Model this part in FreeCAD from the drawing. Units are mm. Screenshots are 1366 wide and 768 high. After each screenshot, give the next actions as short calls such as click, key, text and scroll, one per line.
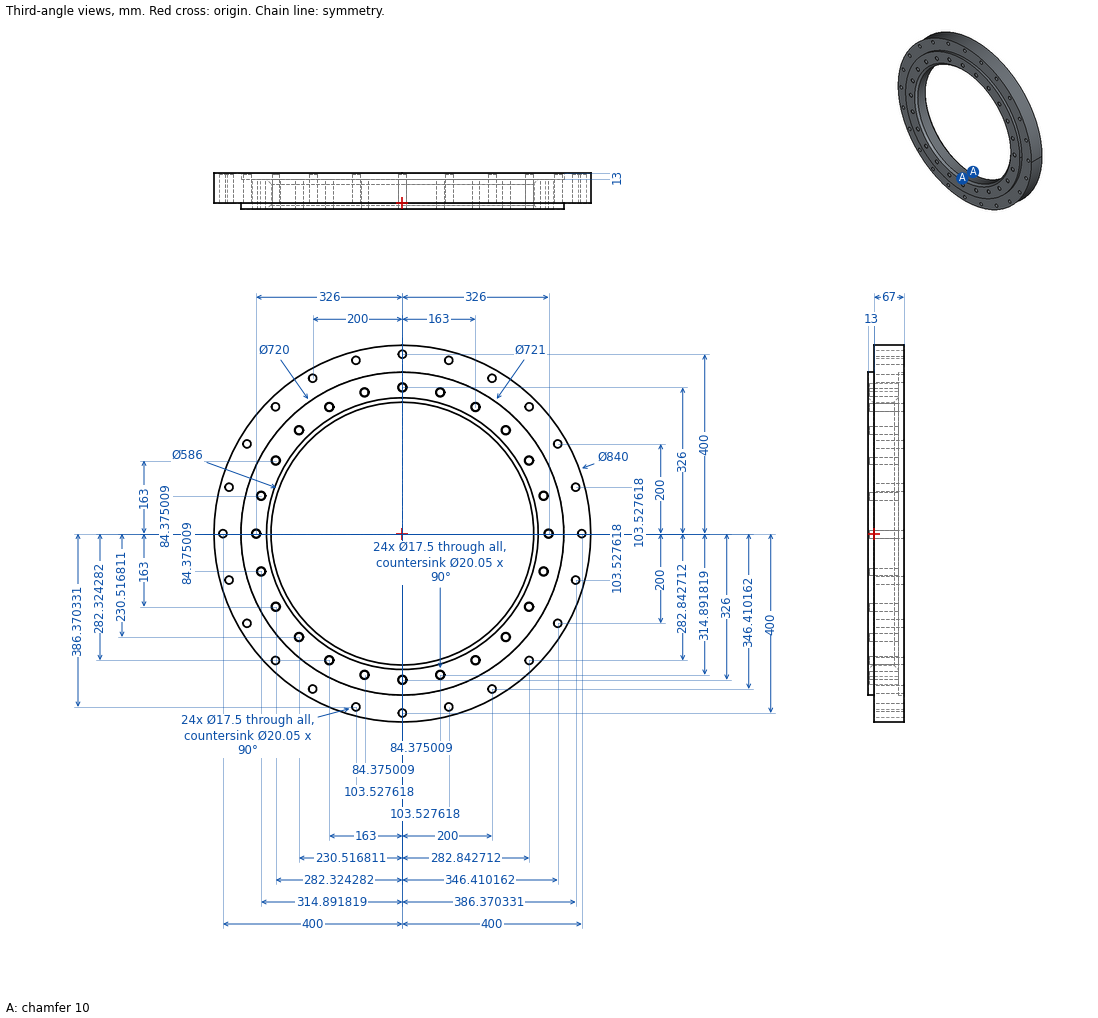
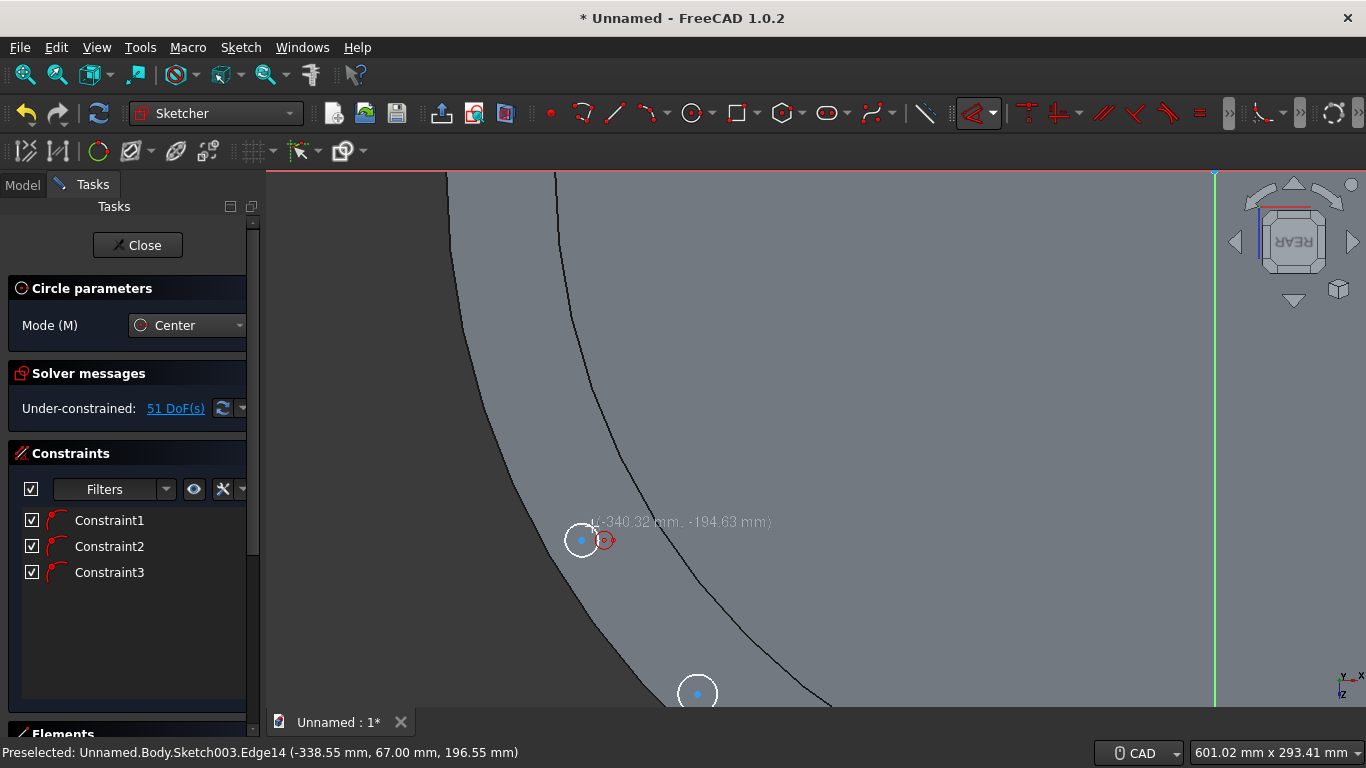
scroll(508, 360, up, 2)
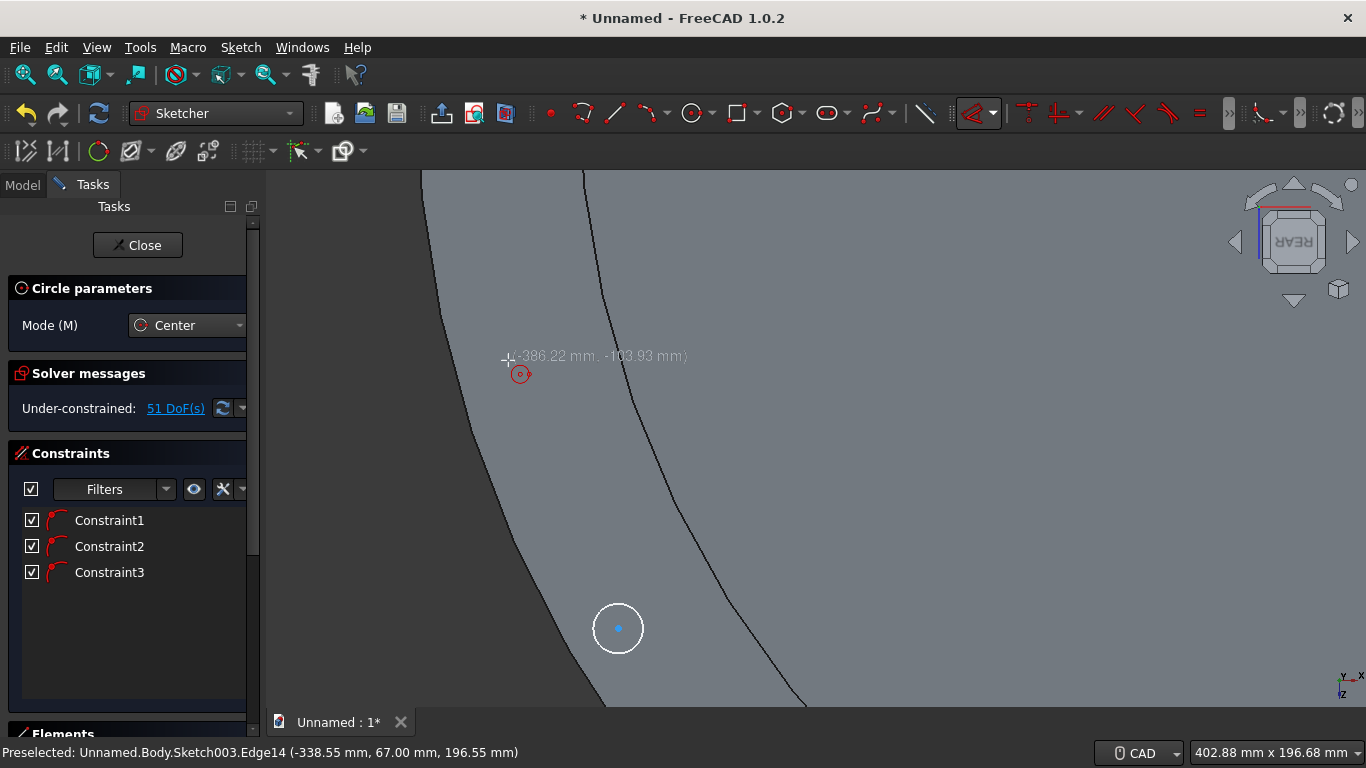
scroll(586, 510, down, 9)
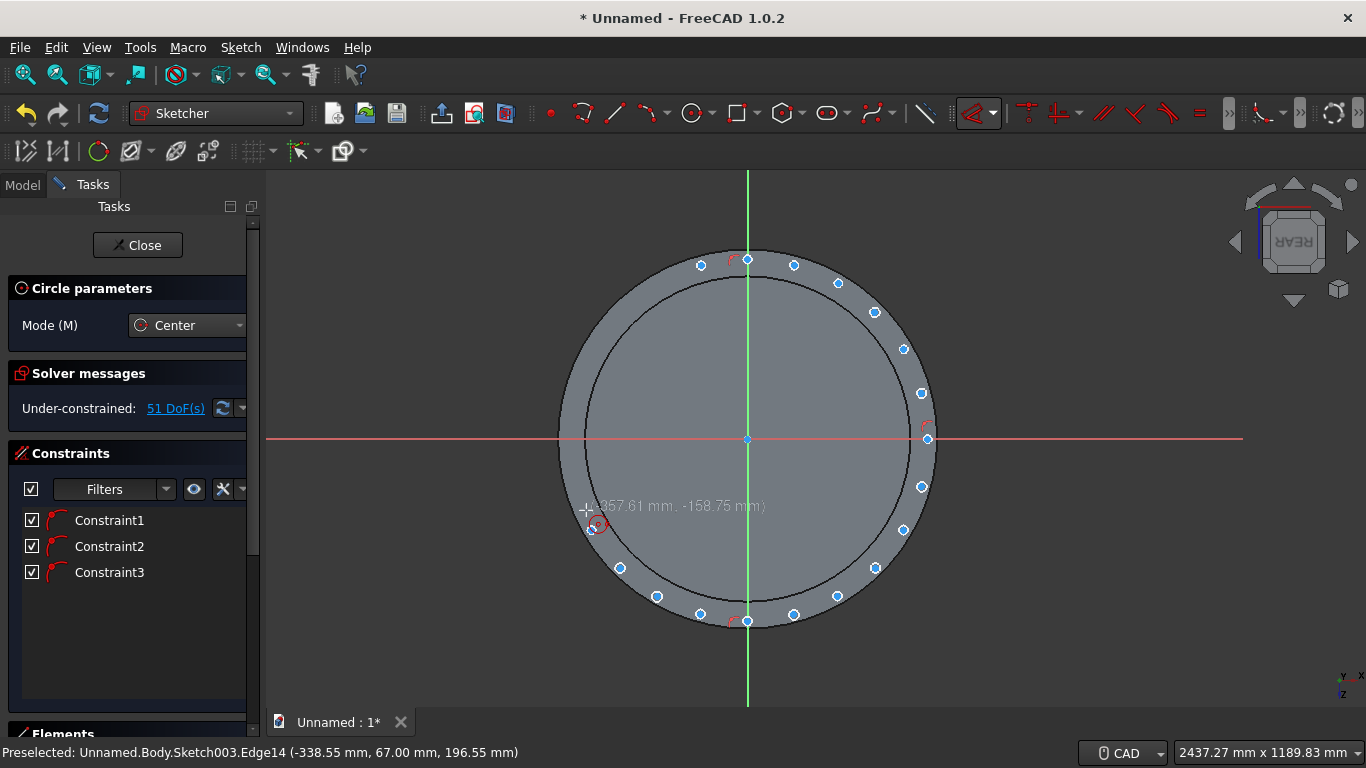
click(573, 486)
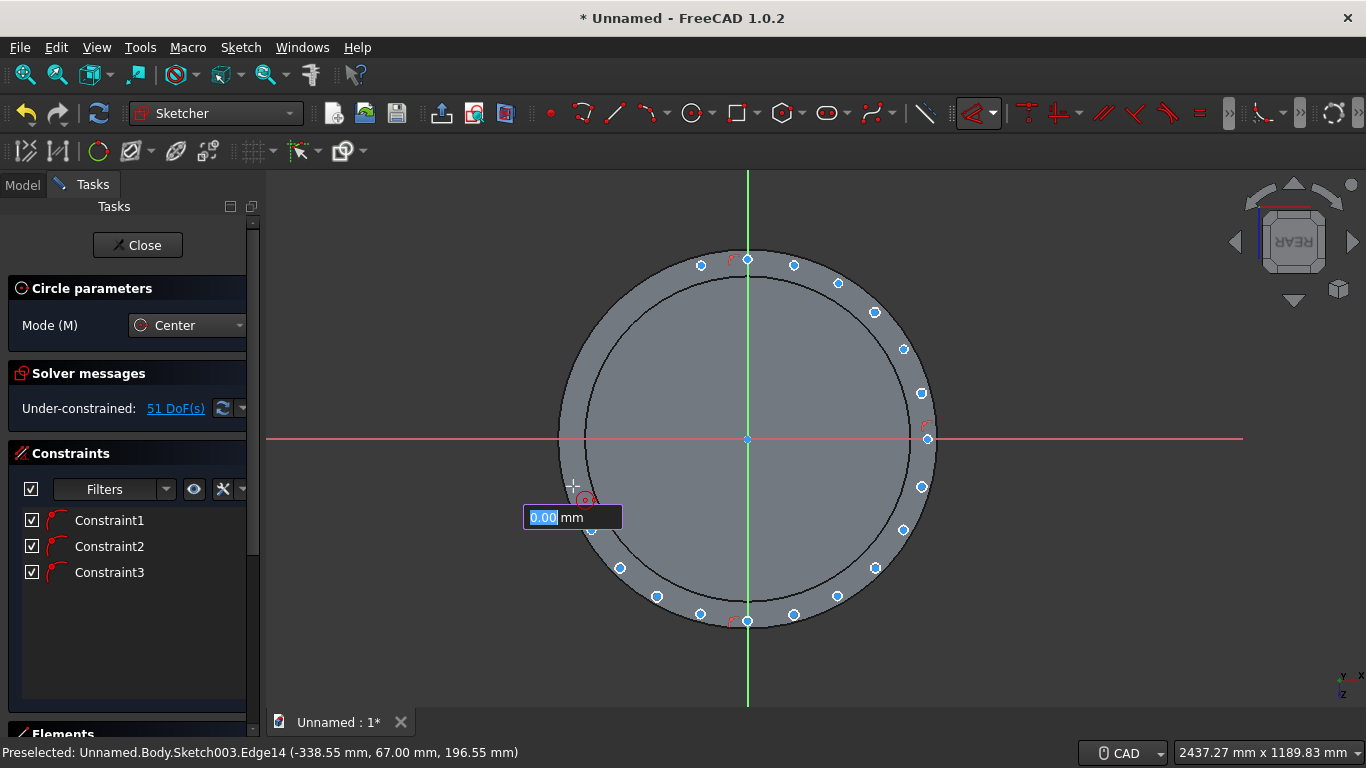
scroll(576, 483, up, 7)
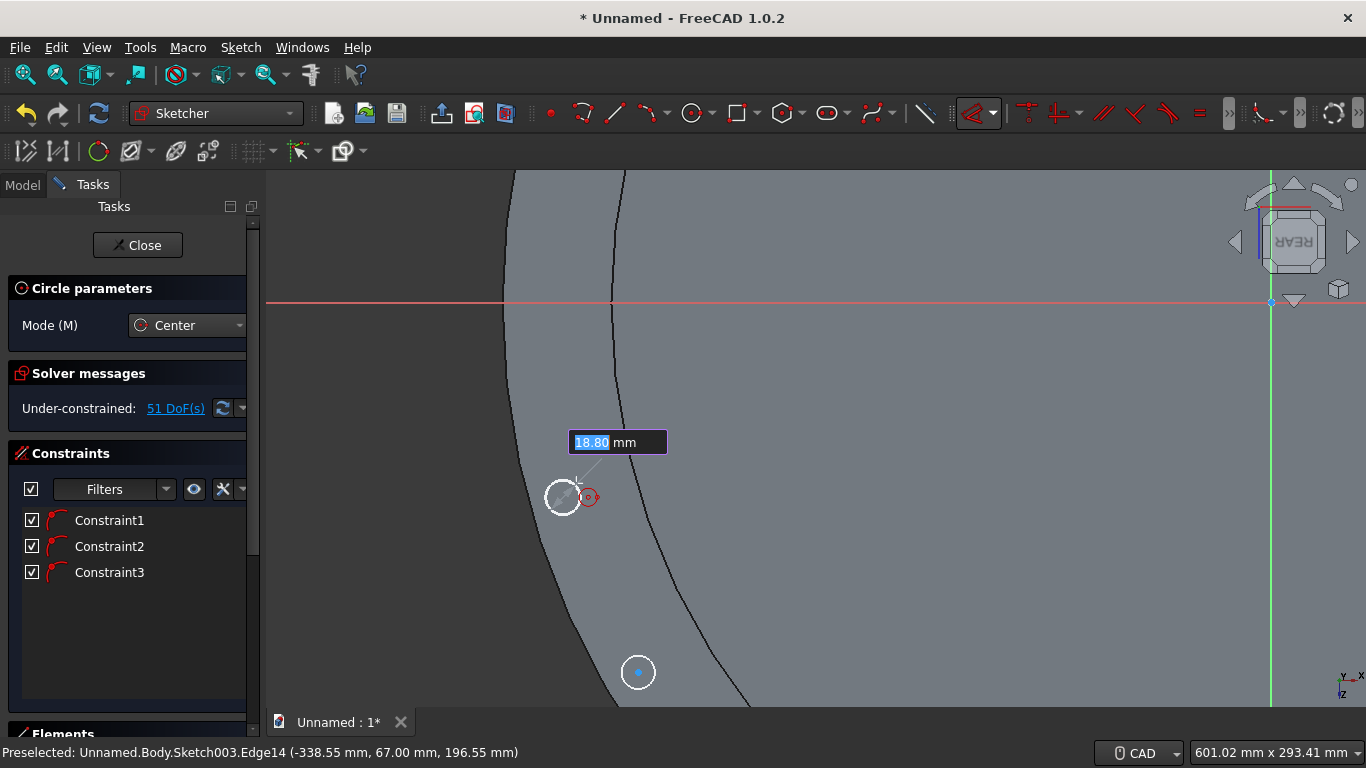
click(575, 481)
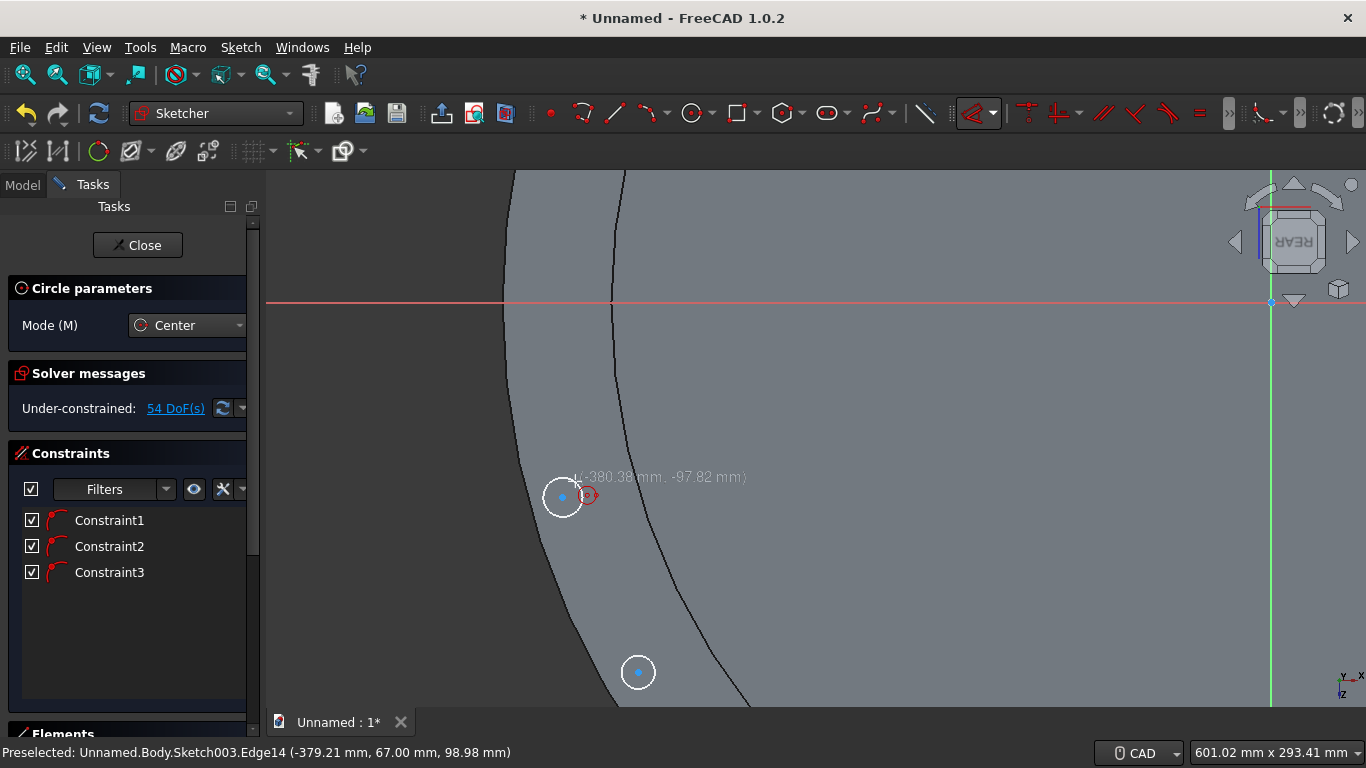
scroll(539, 303, up, 2)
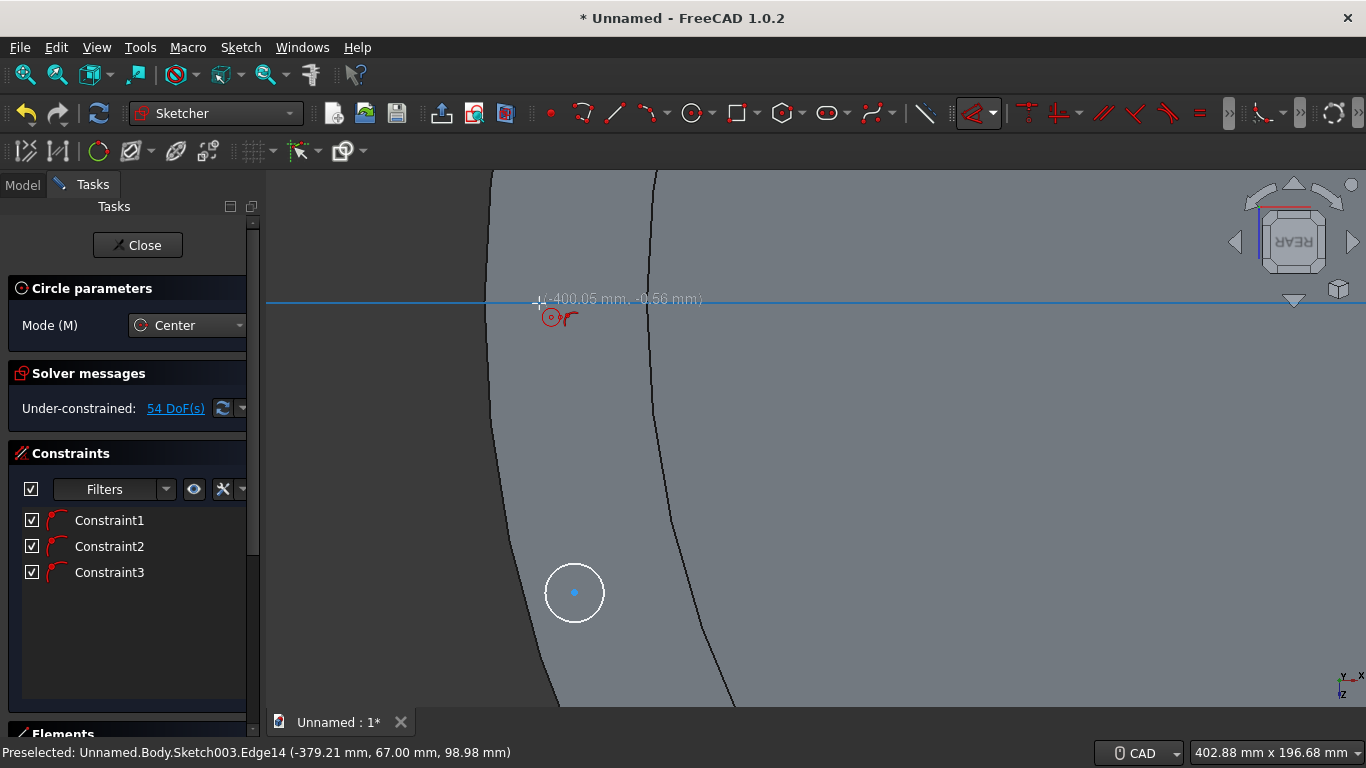
scroll(573, 465, down, 9)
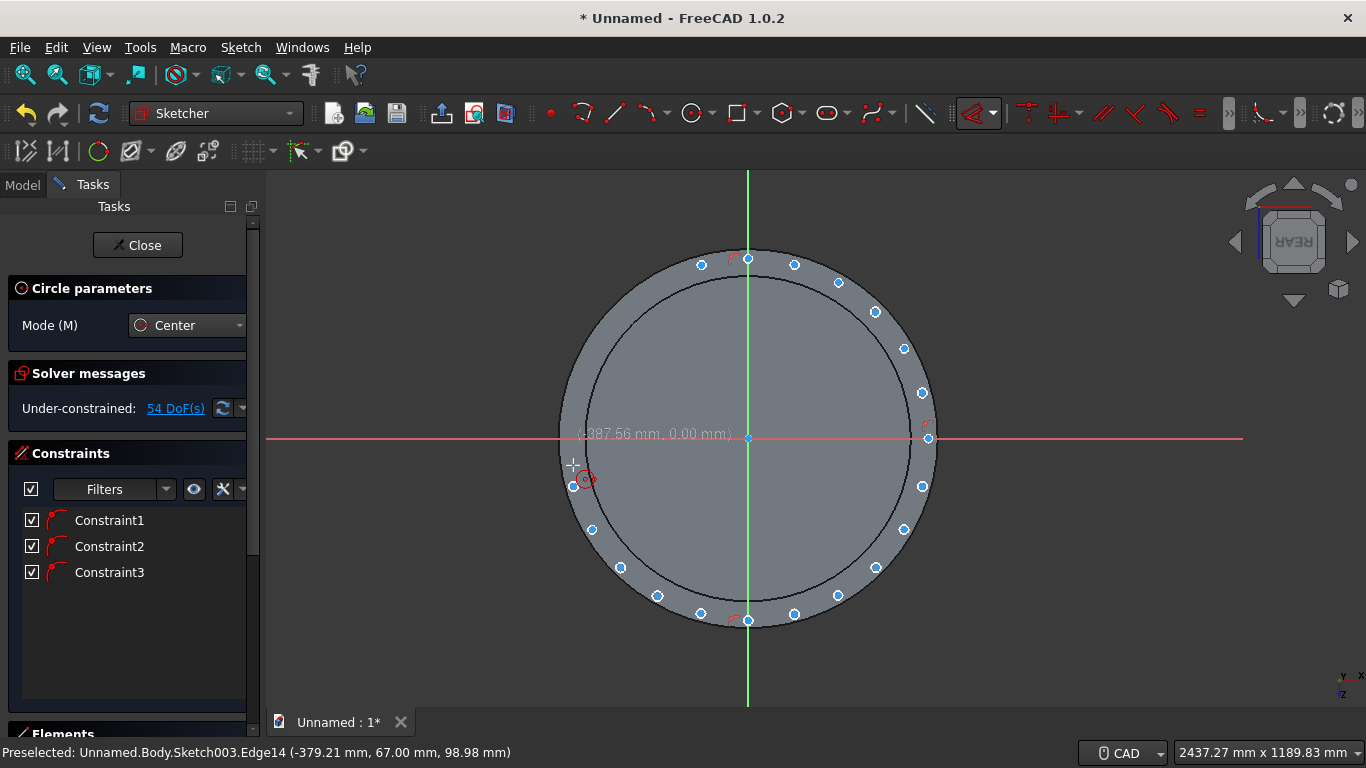
click(568, 439)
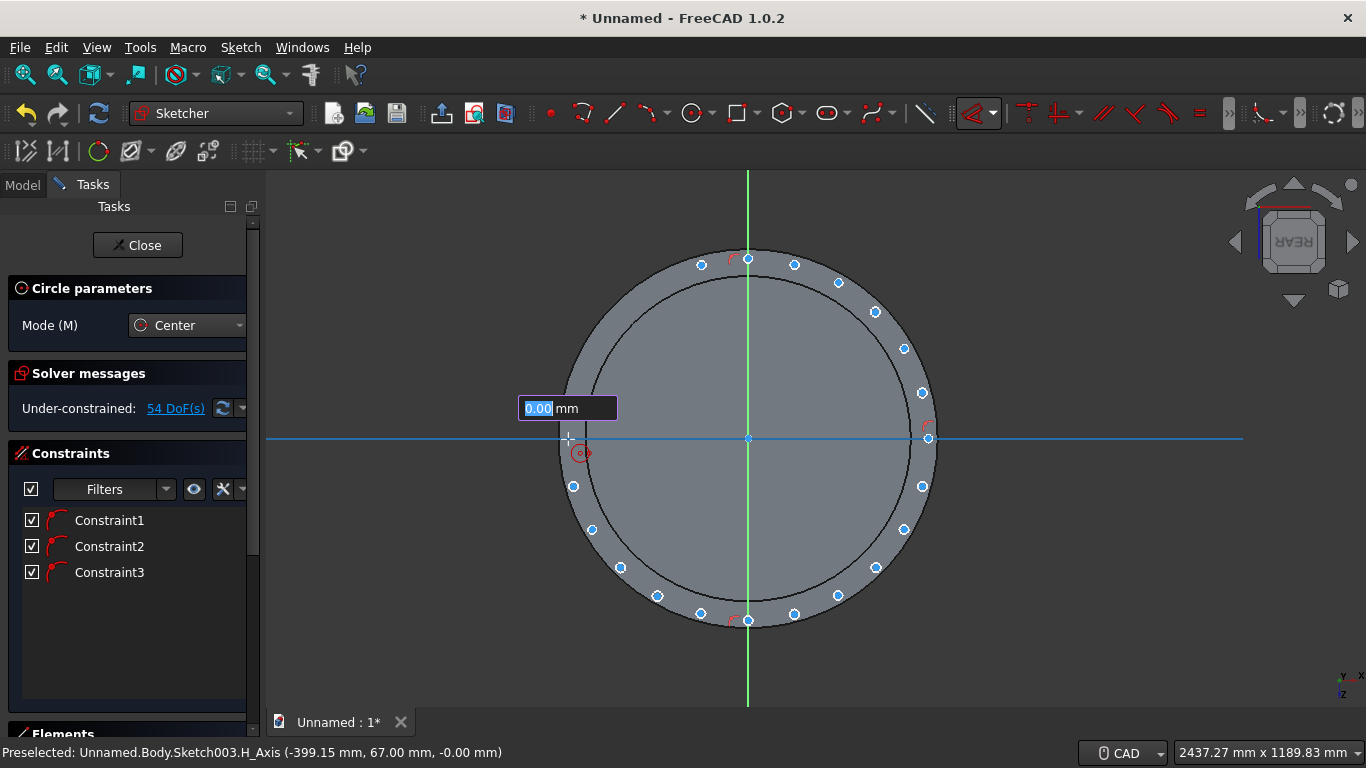
scroll(569, 435, up, 8)